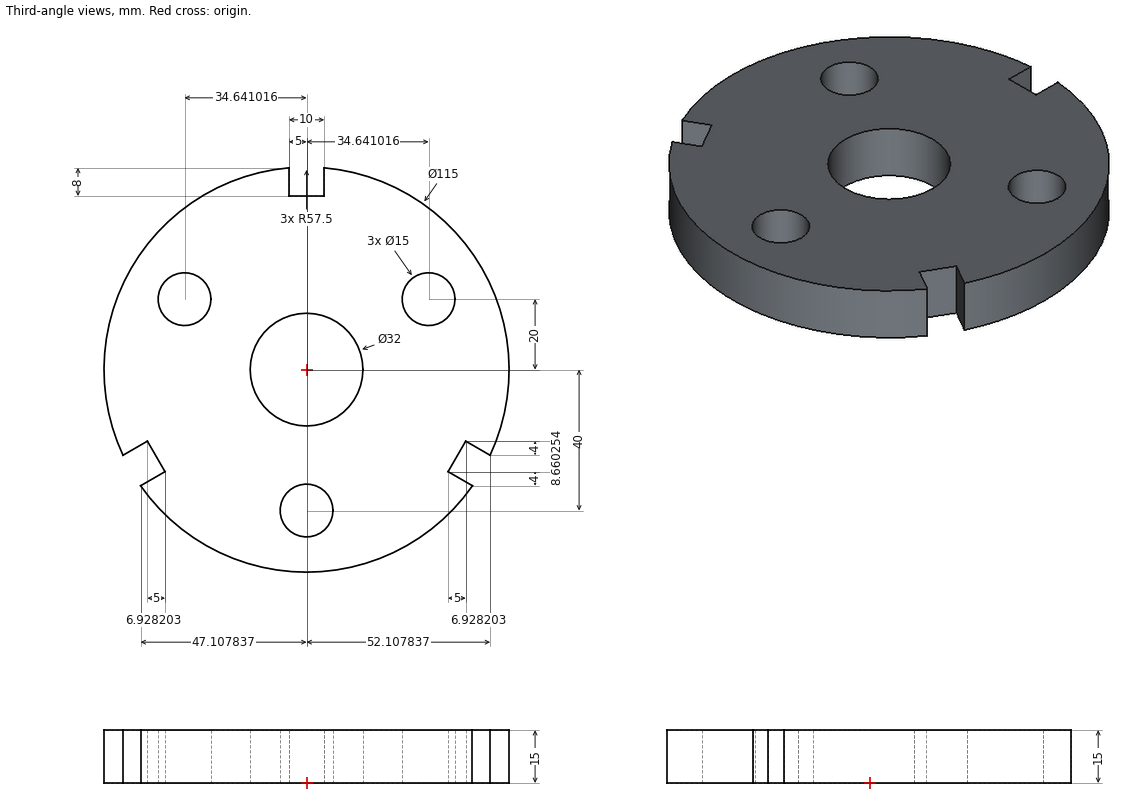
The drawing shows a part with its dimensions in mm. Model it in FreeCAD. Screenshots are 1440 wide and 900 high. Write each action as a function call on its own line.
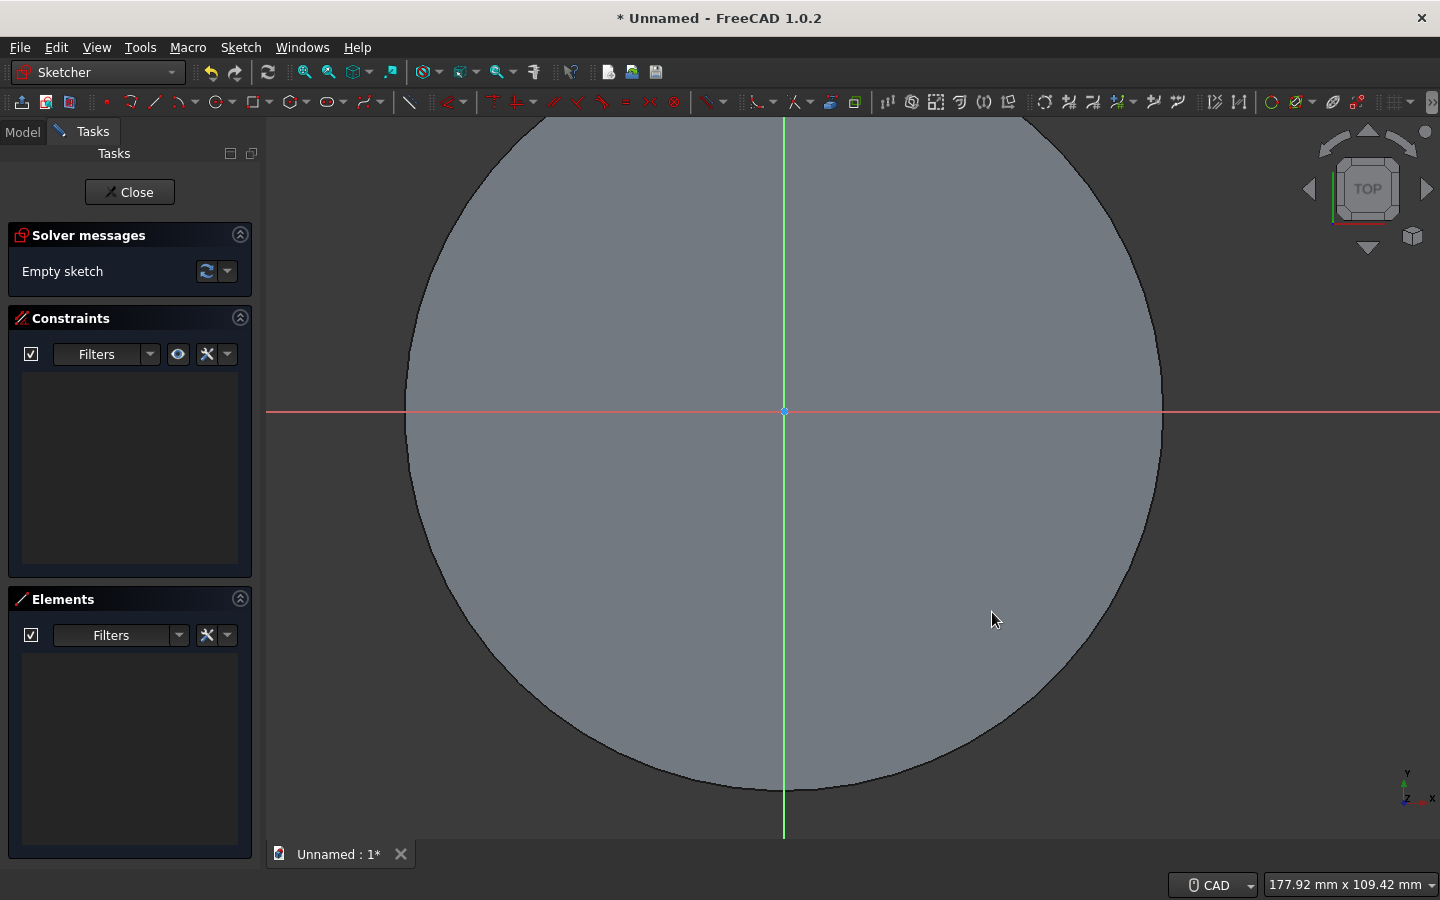
click(216, 102)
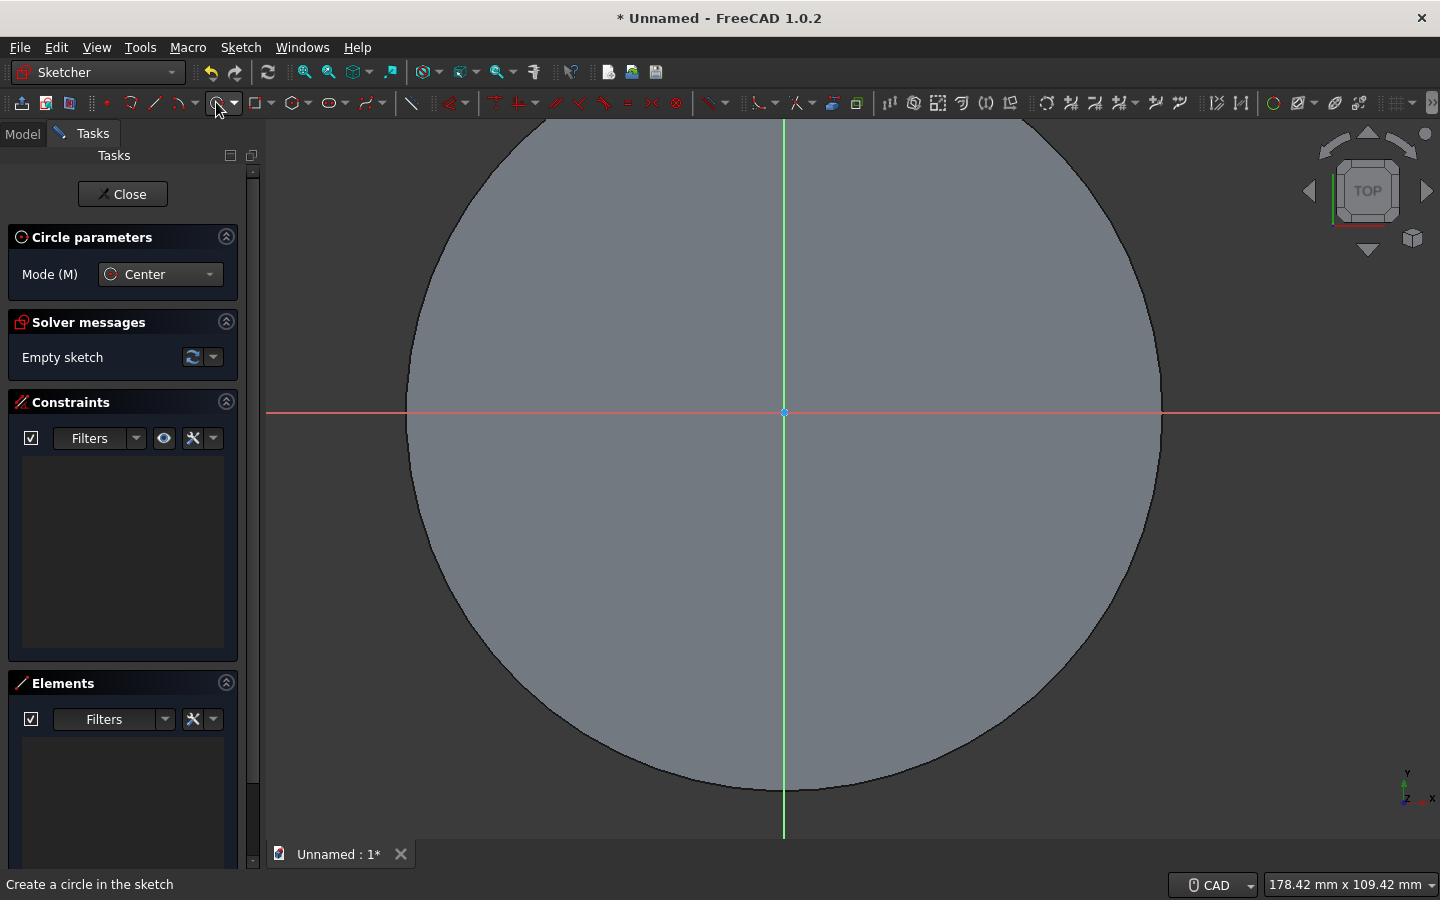
click(1012, 281)
move(1047, 246)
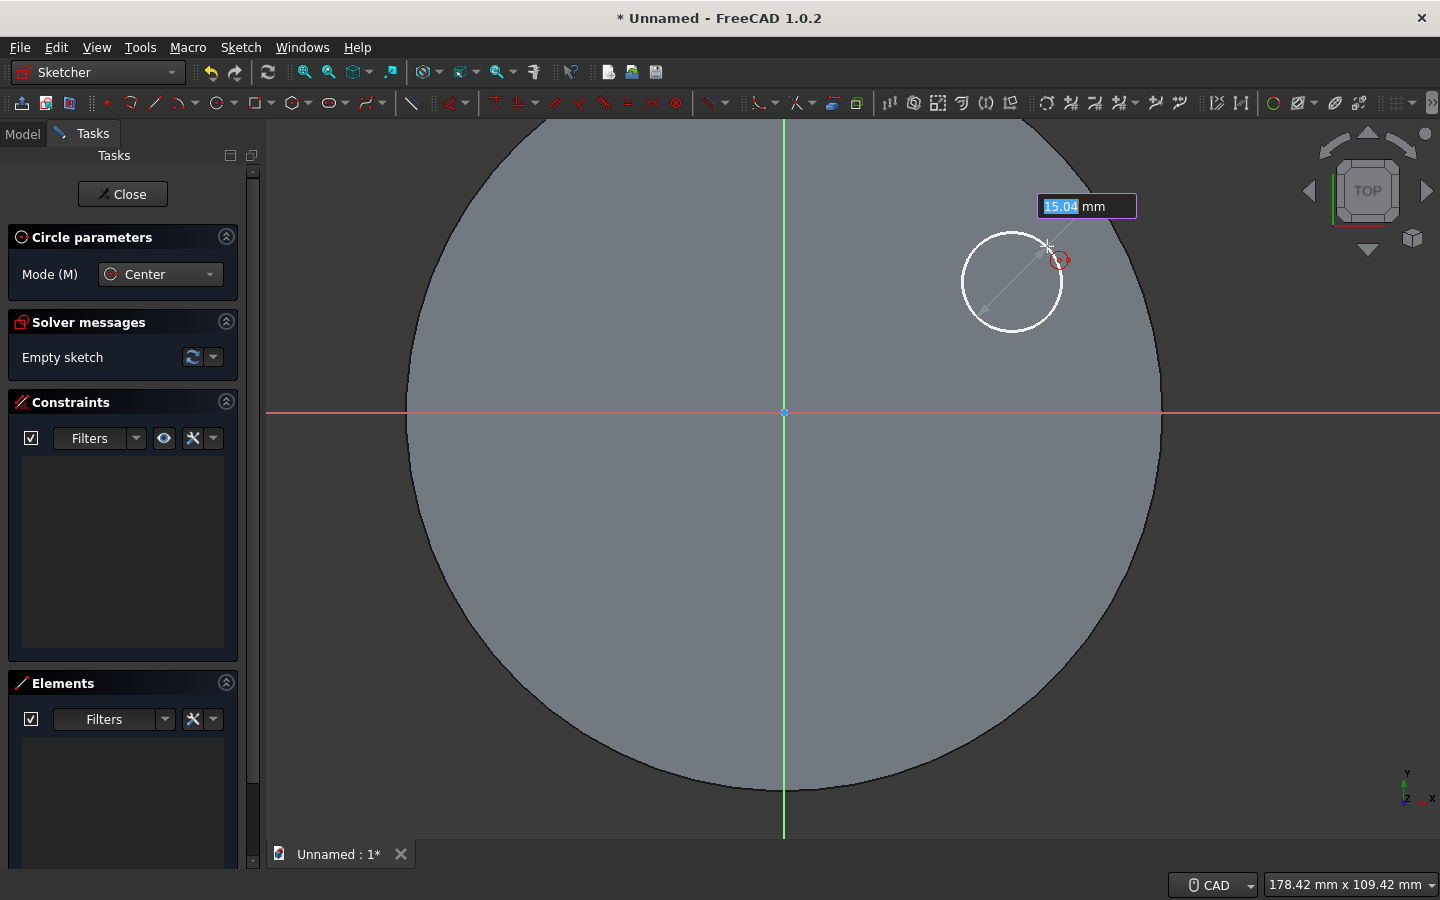
text(15)
key(Return)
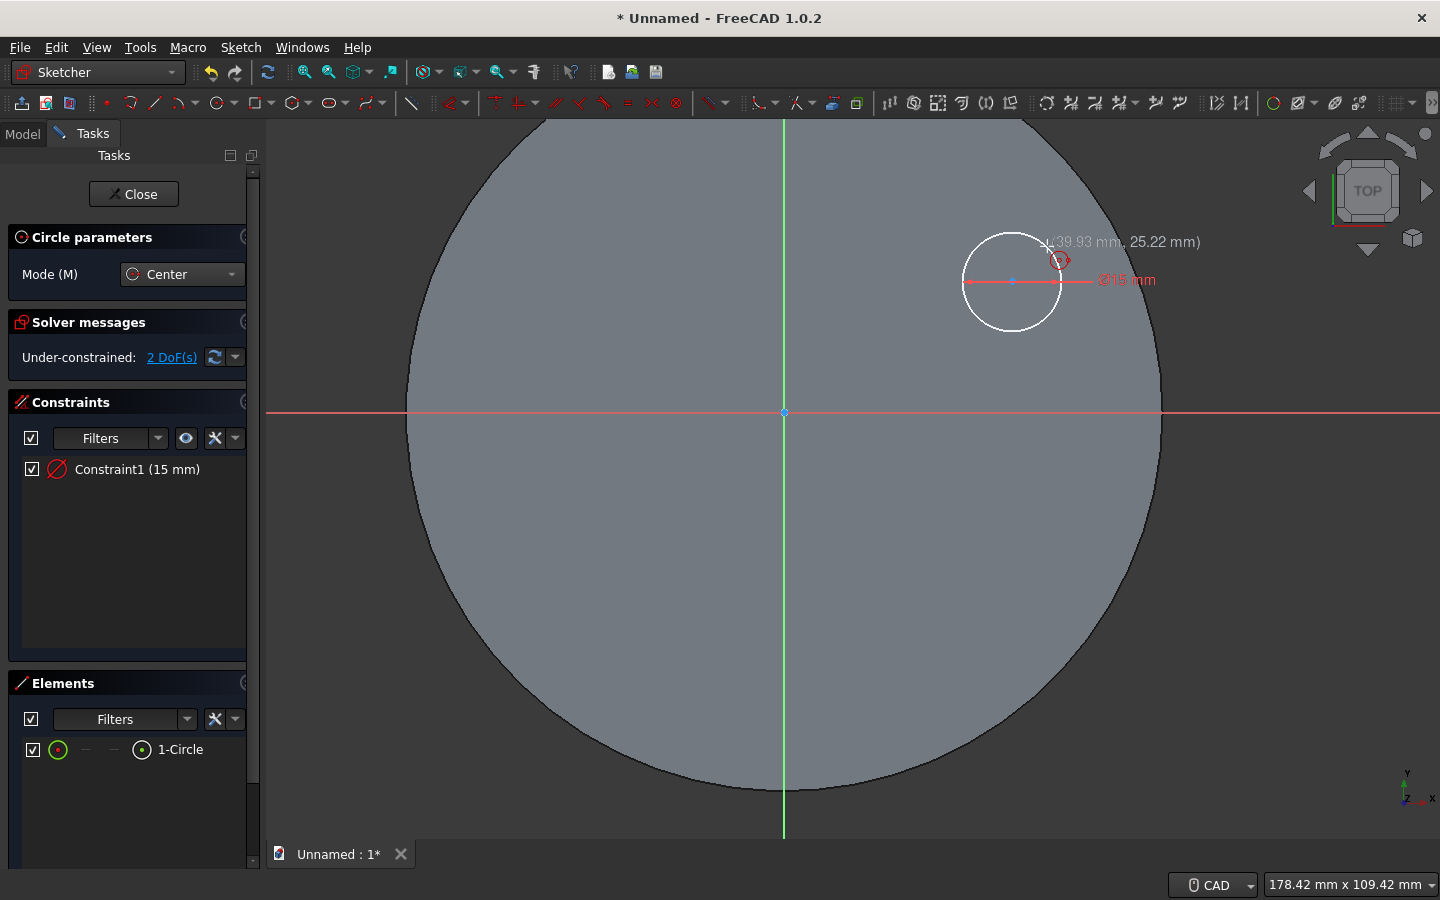
click(784, 676)
move(819, 641)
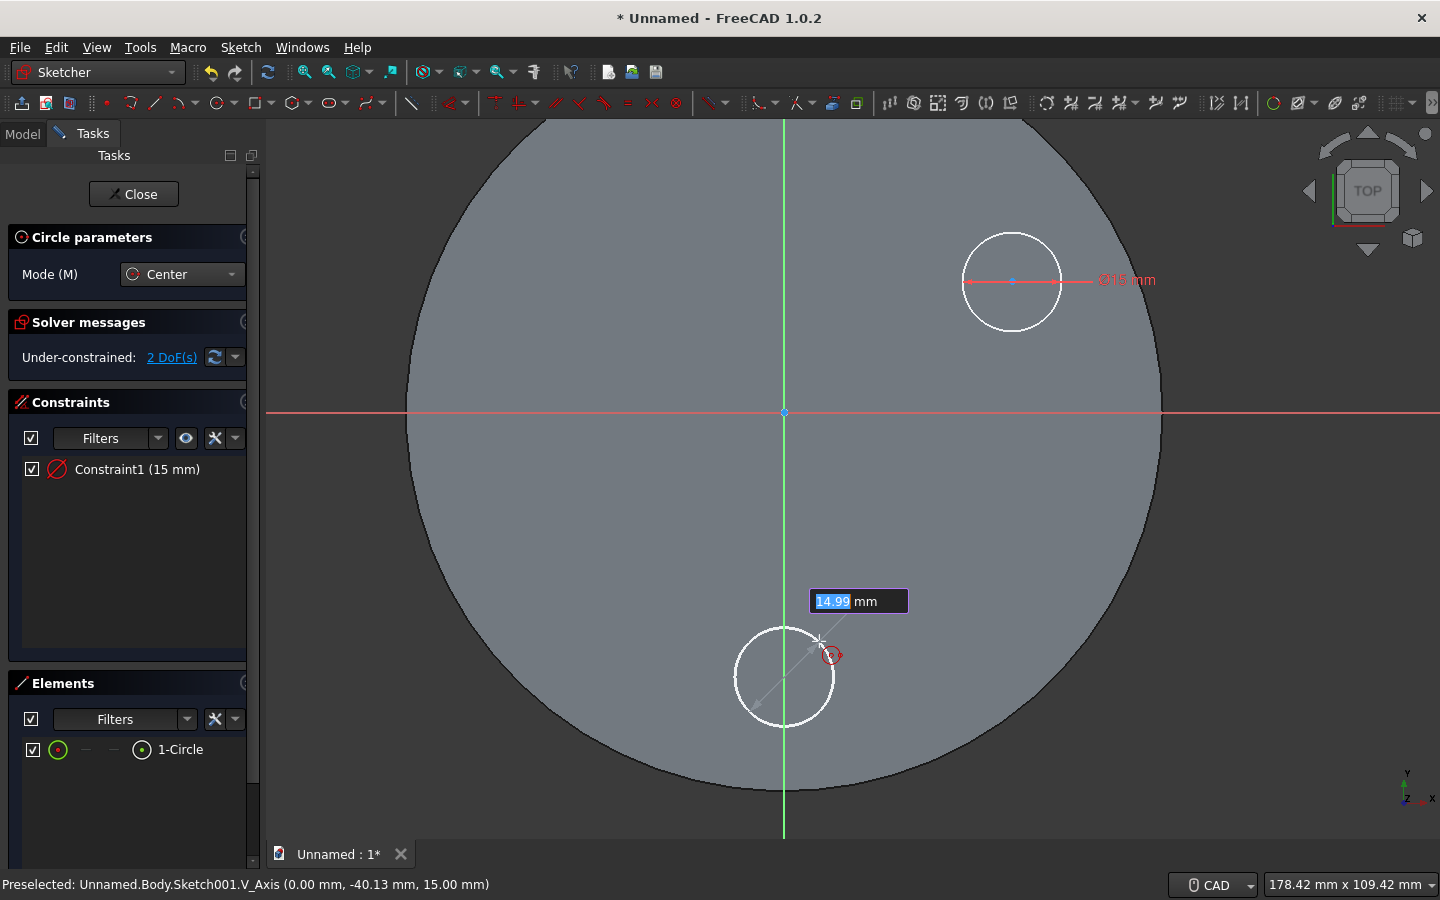
text(15)
key(Return)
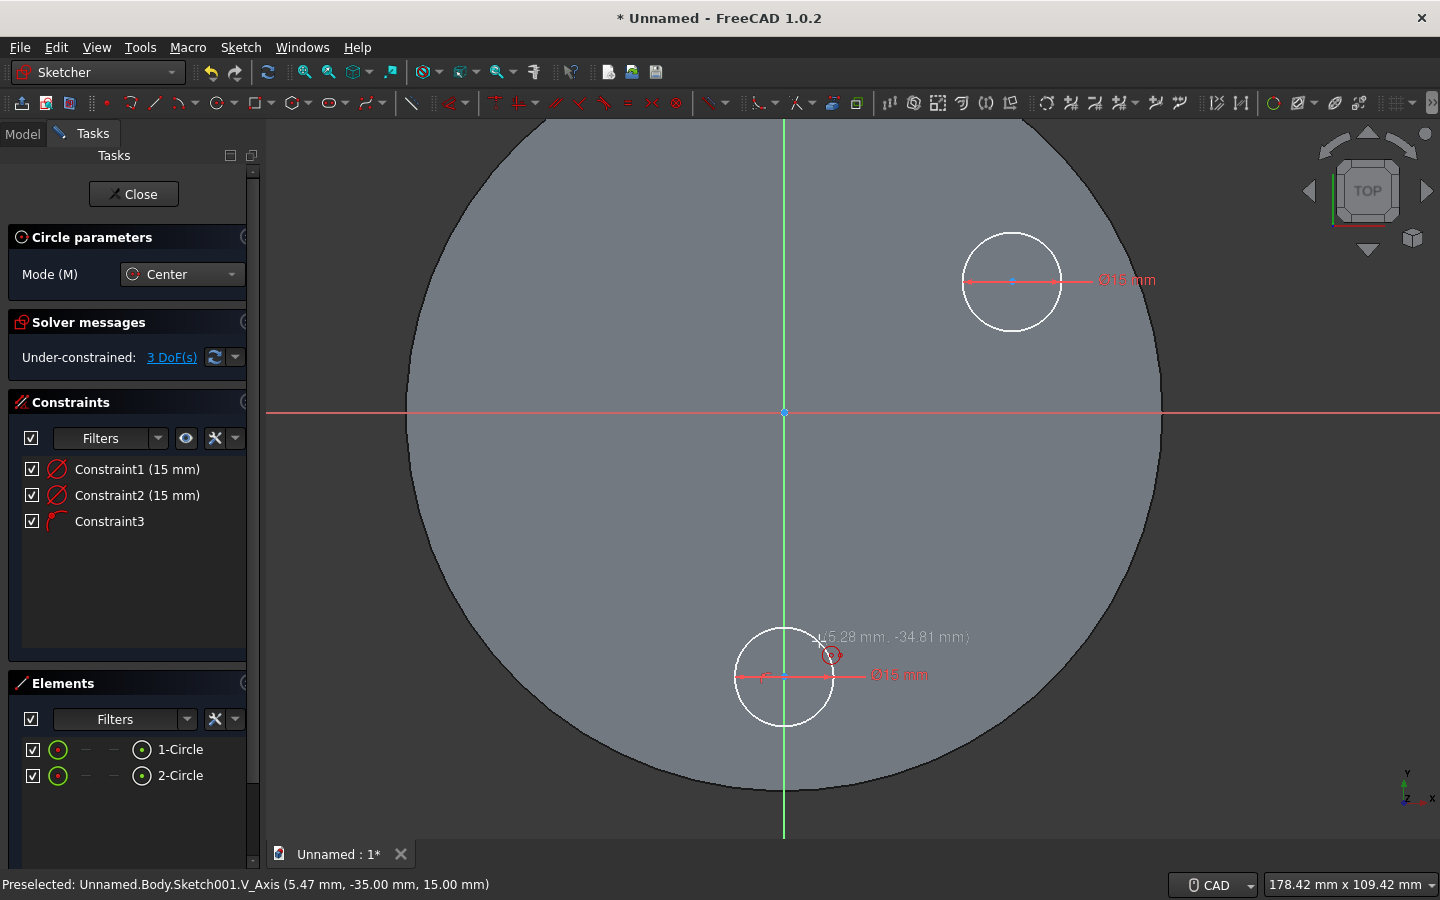
click(556, 281)
move(591, 246)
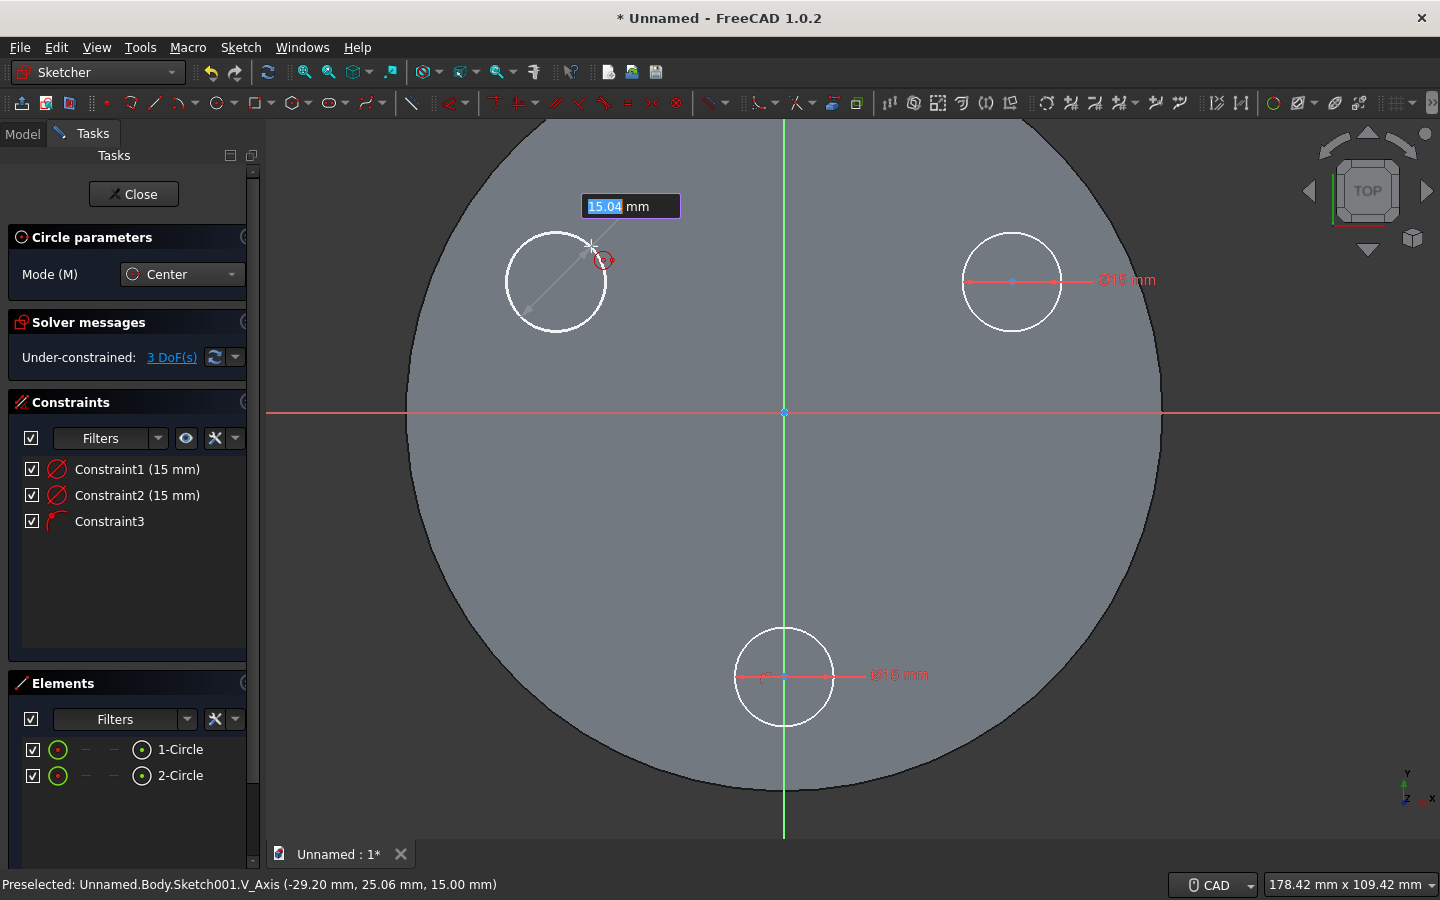
text(15)
key(Return)
key(Escape)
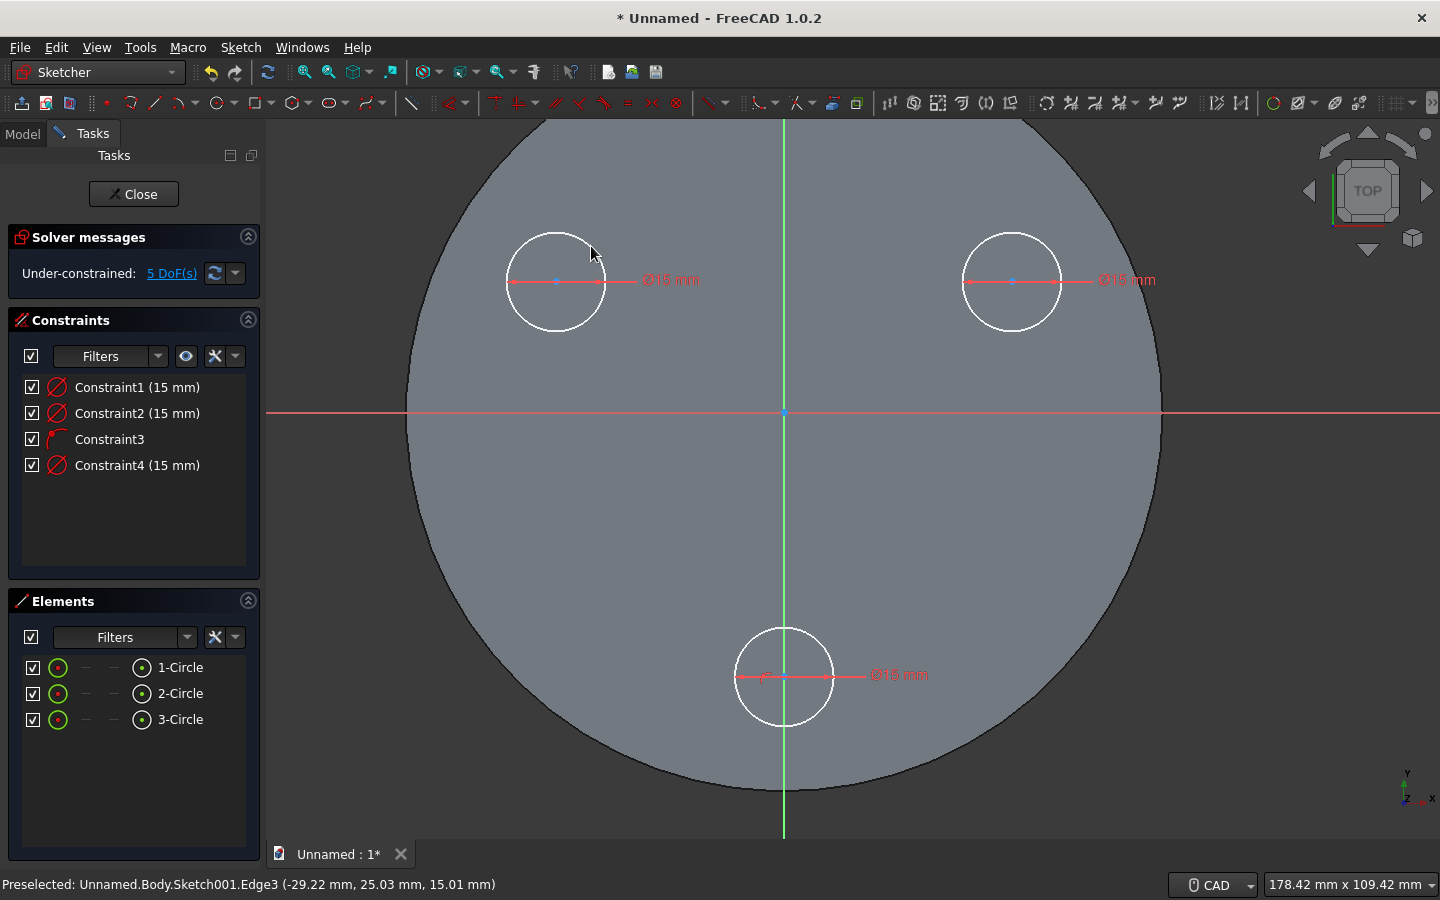
click(1012, 282)